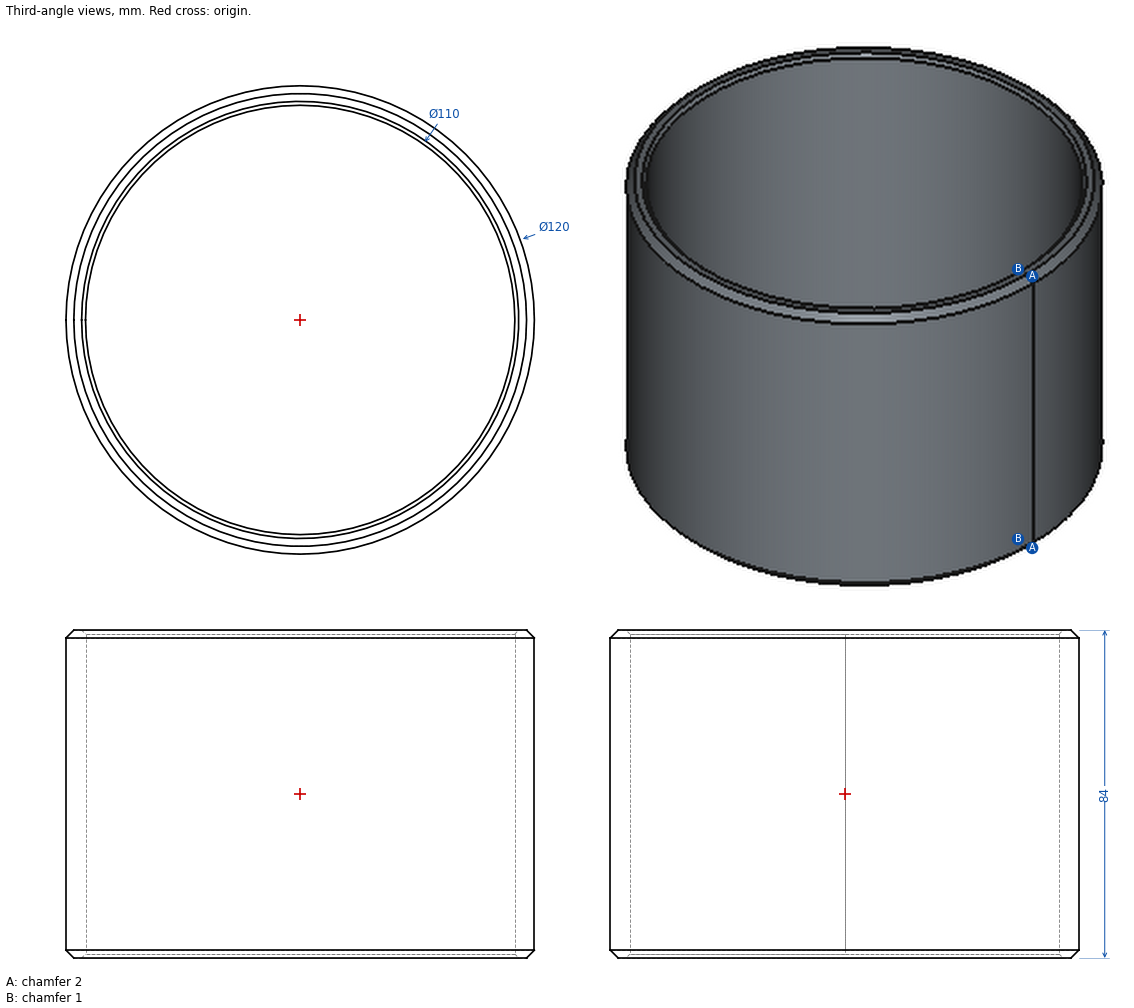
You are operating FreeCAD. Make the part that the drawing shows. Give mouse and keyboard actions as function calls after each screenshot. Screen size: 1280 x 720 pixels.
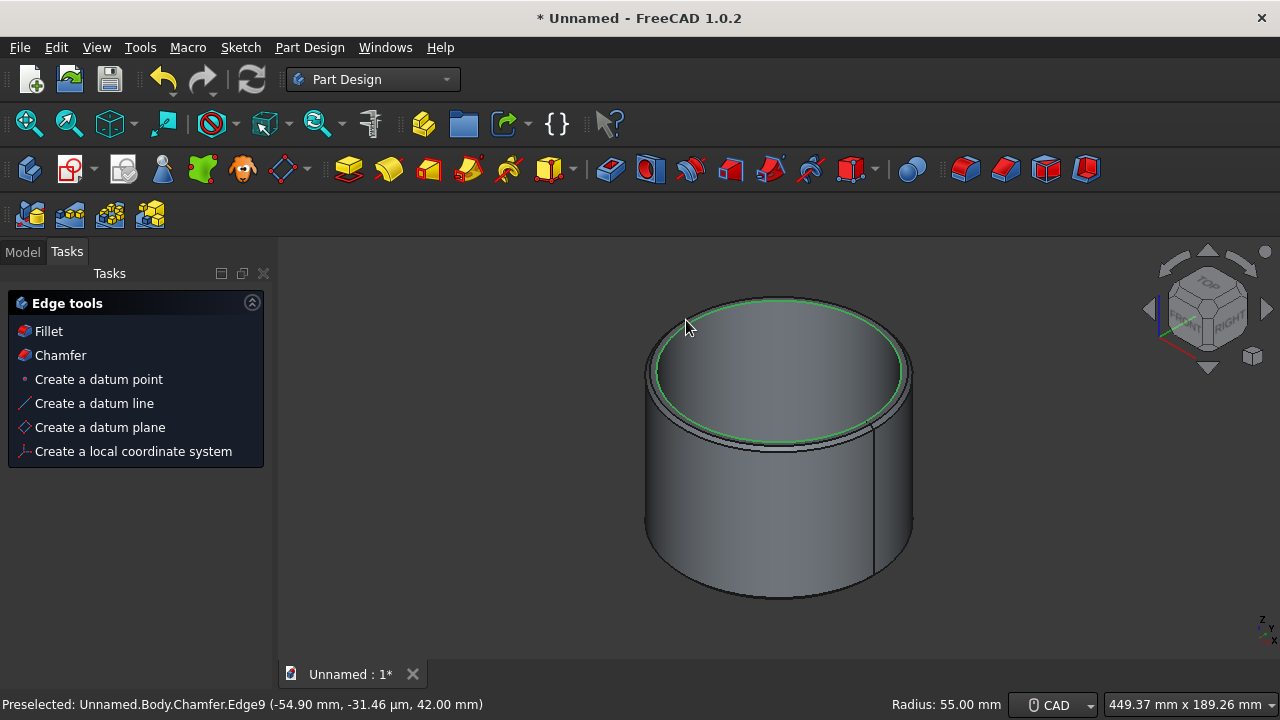
key(2)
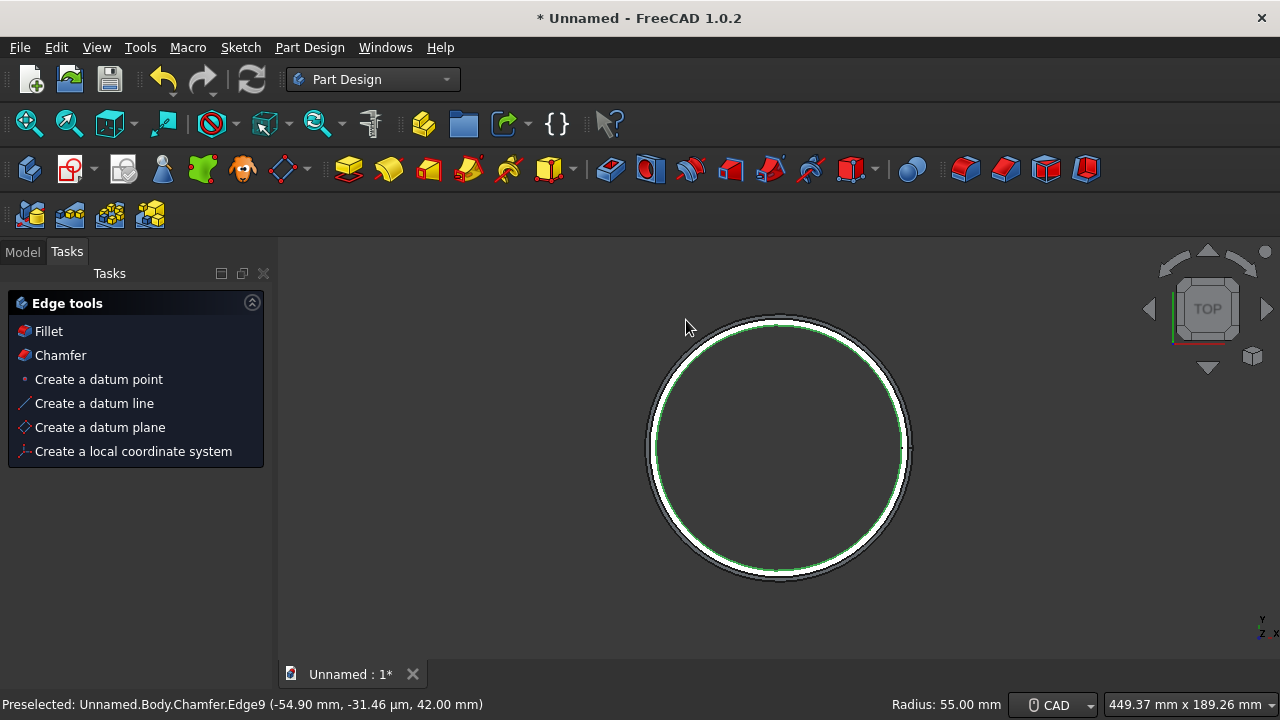
key(1)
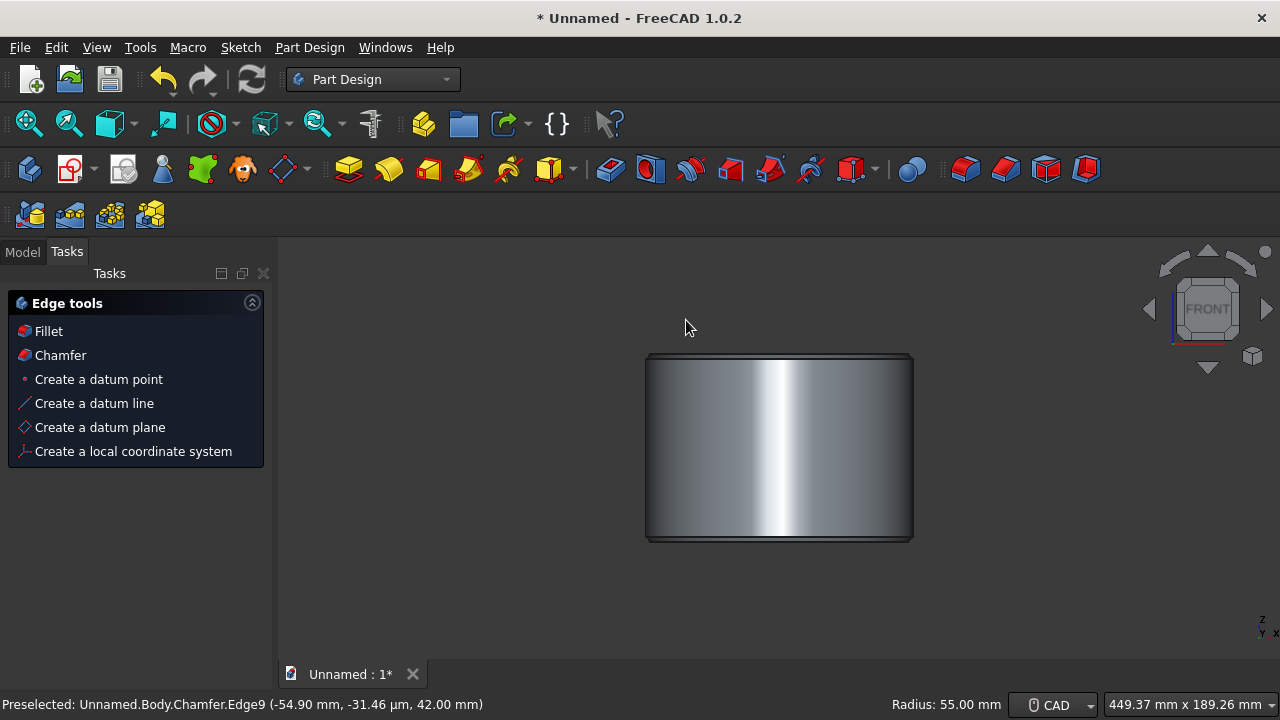
click(30, 124)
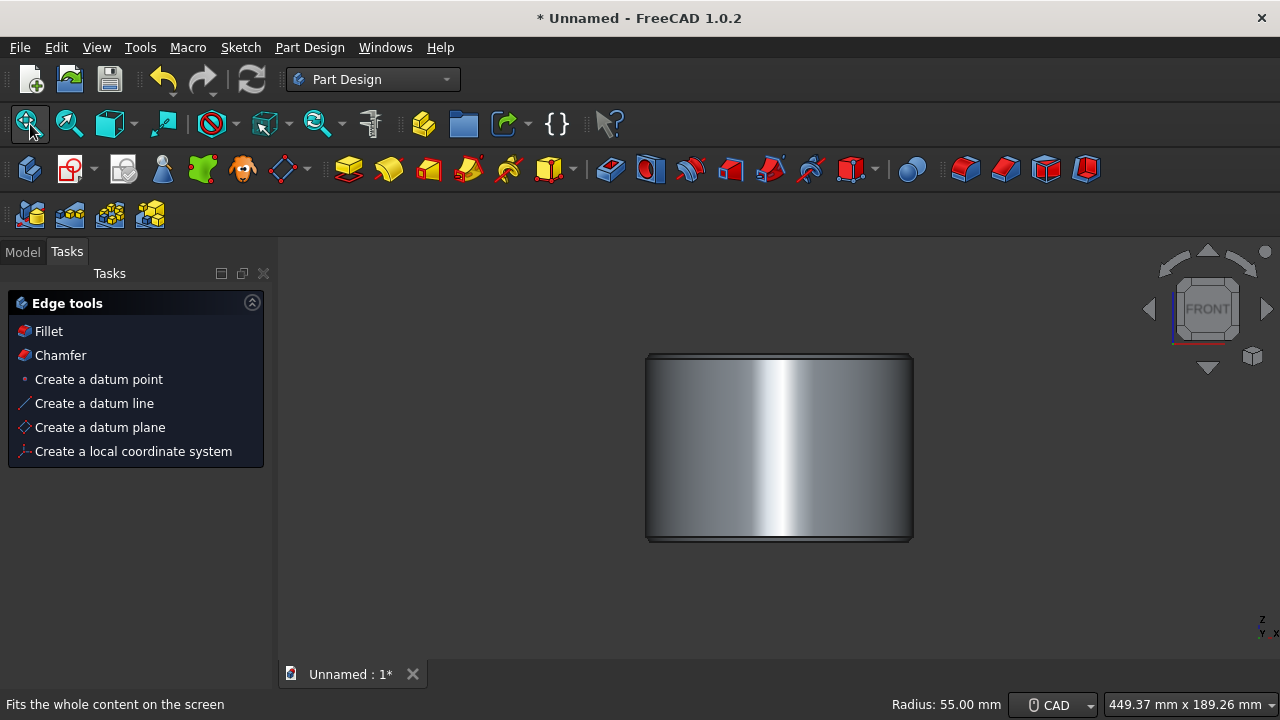
key(3)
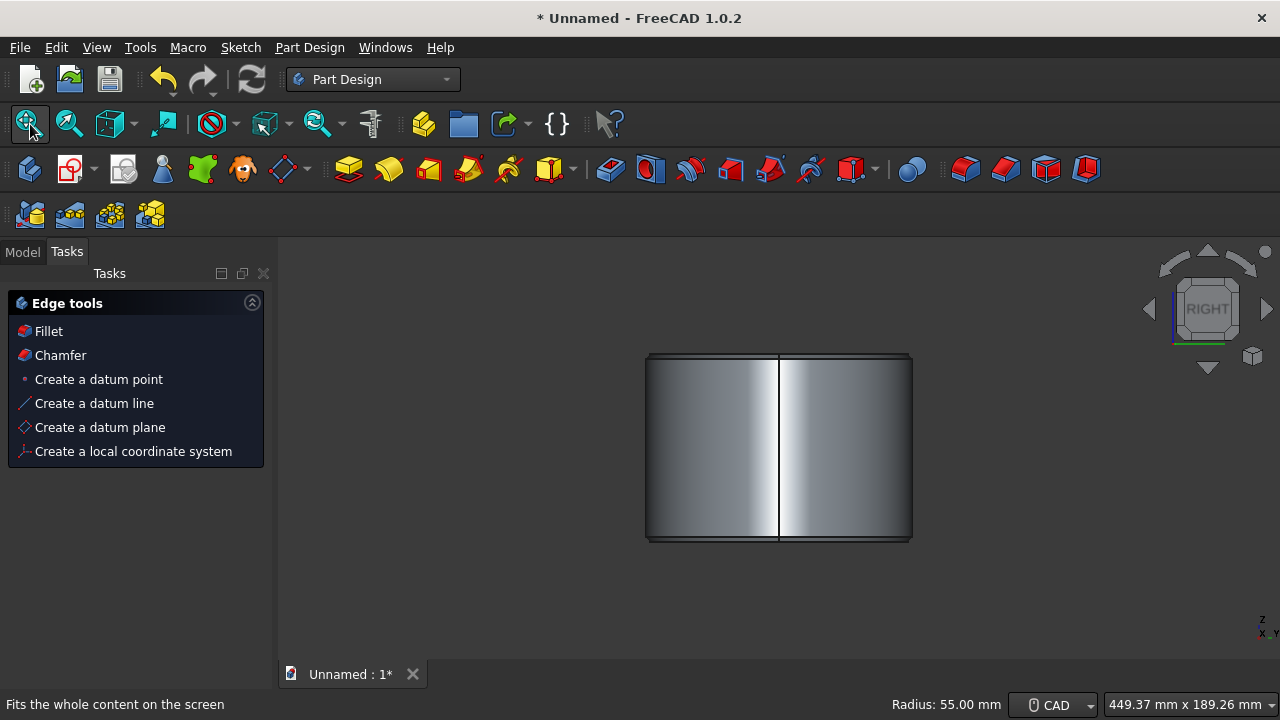
click(30, 124)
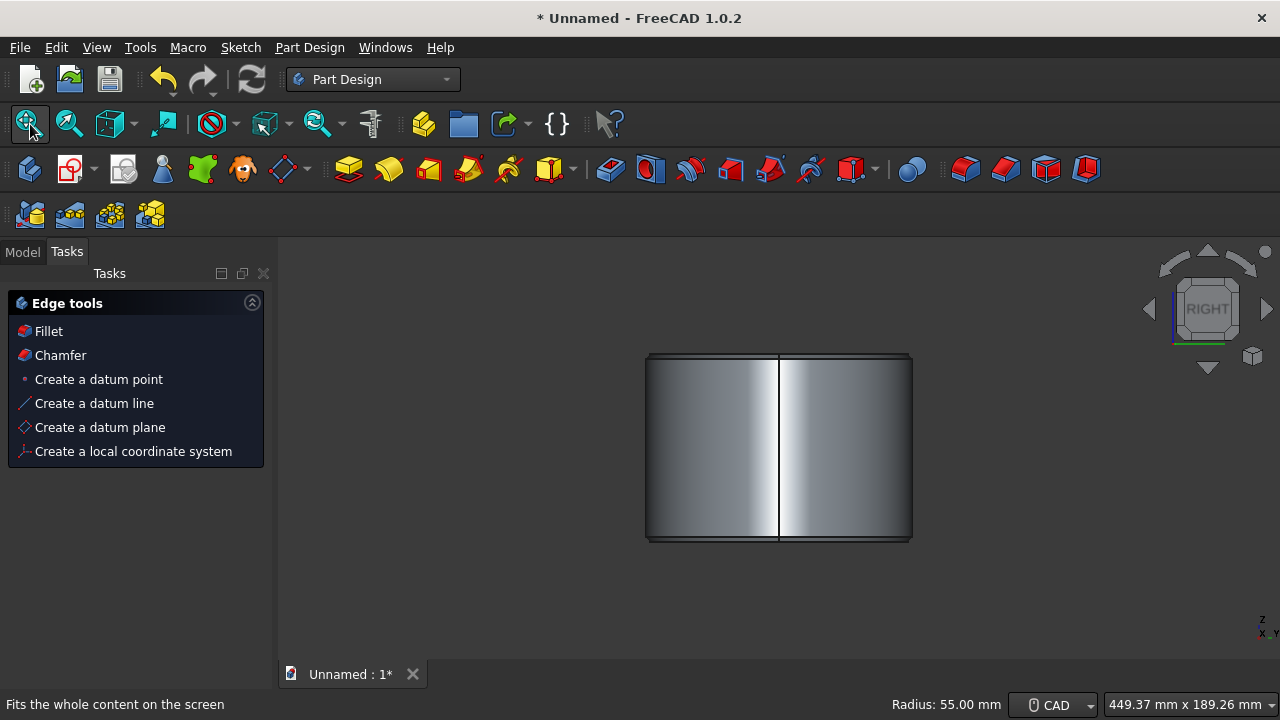
key(5)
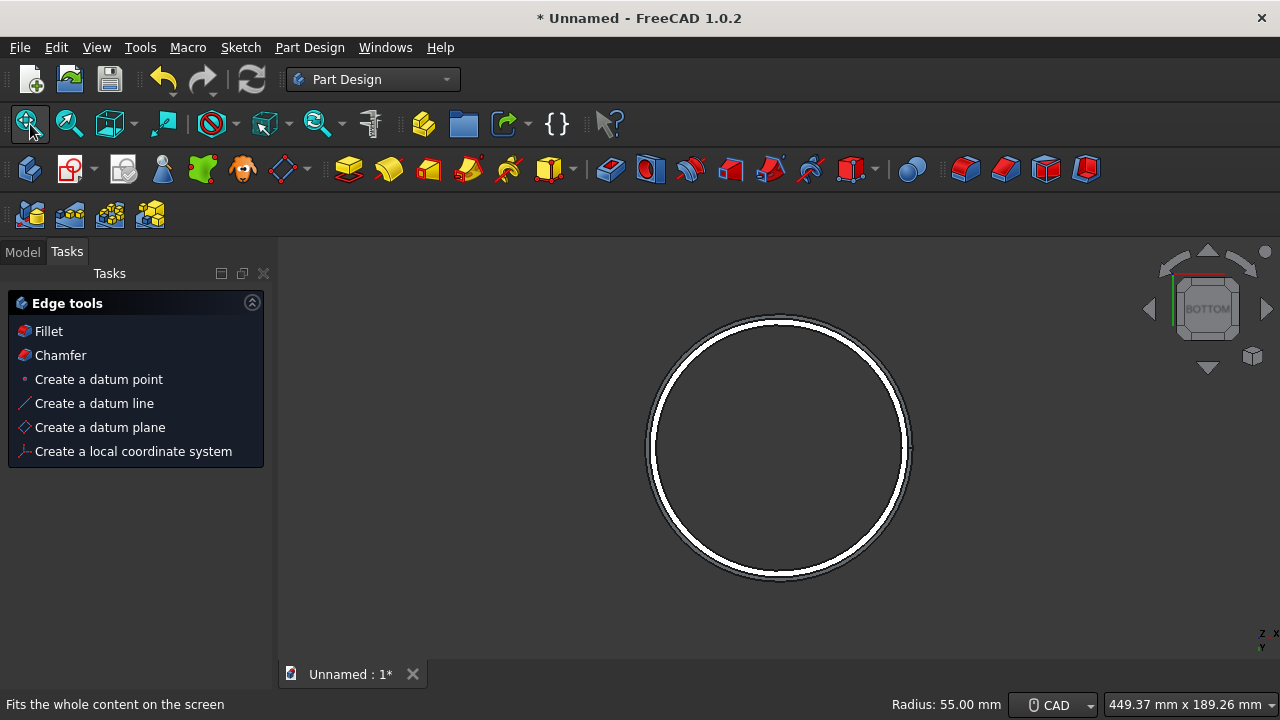
click(656, 447, ctrl)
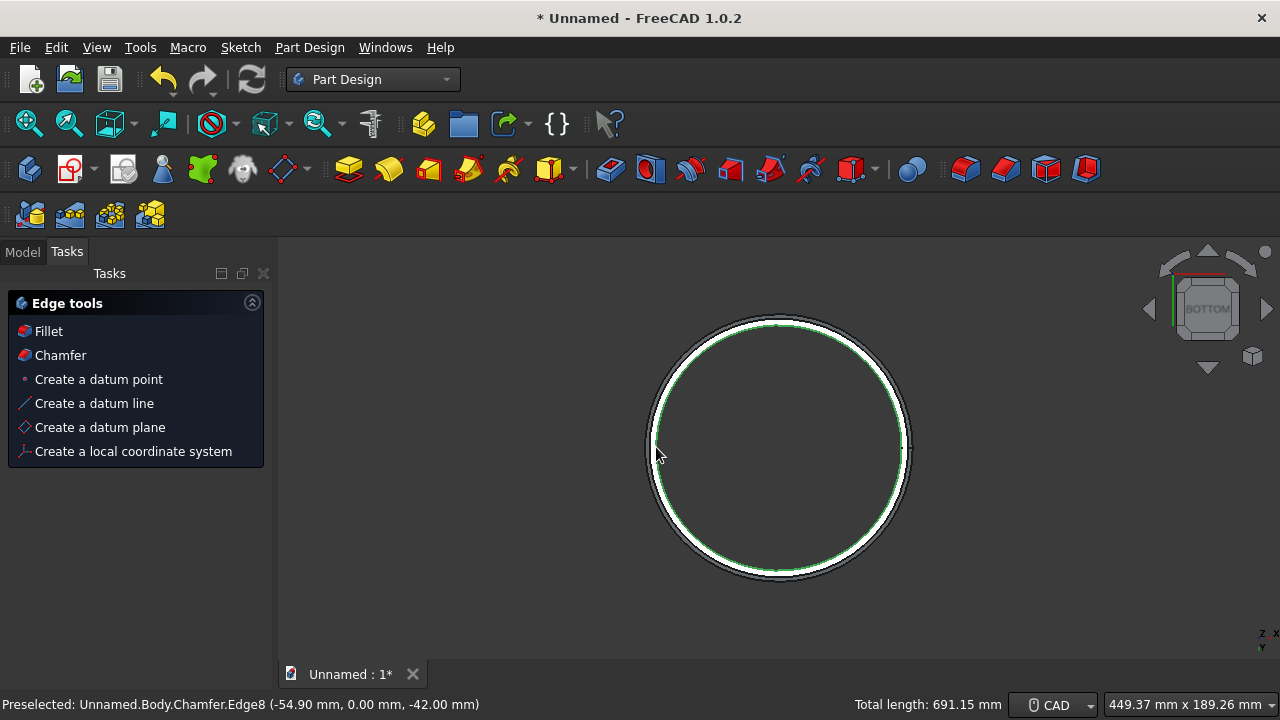
click(1006, 170)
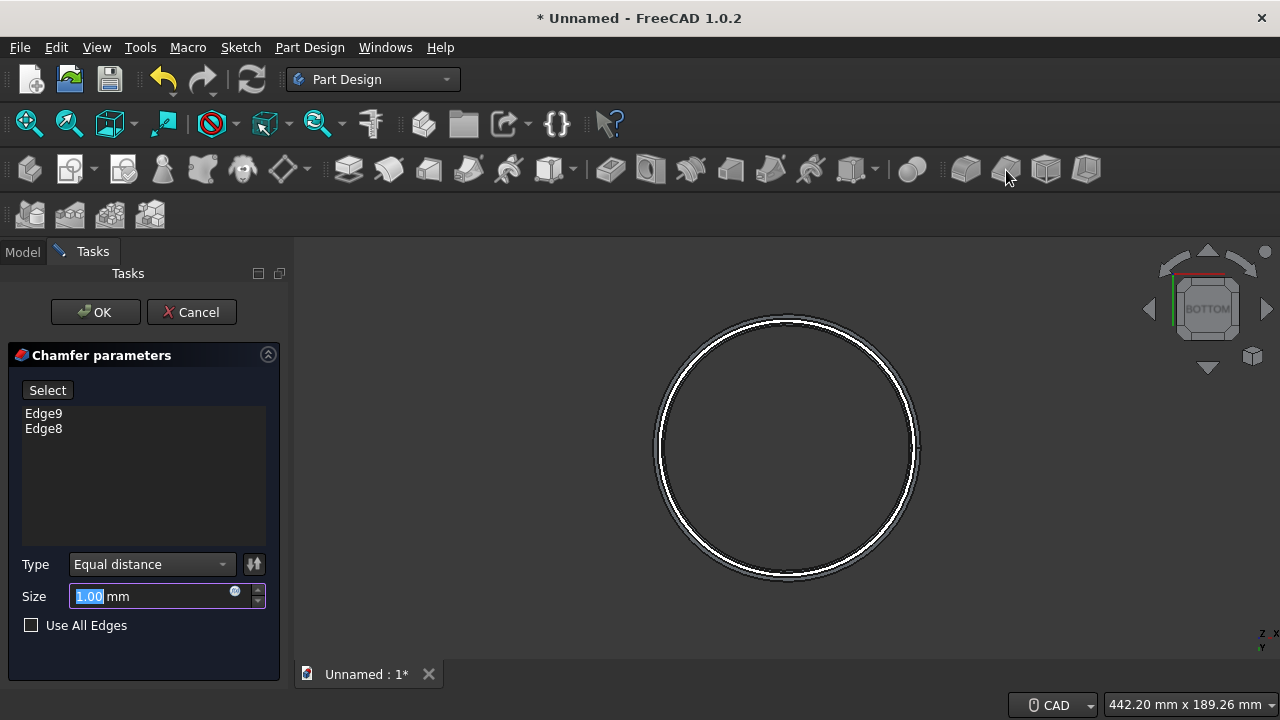
text(1)
key(Tab)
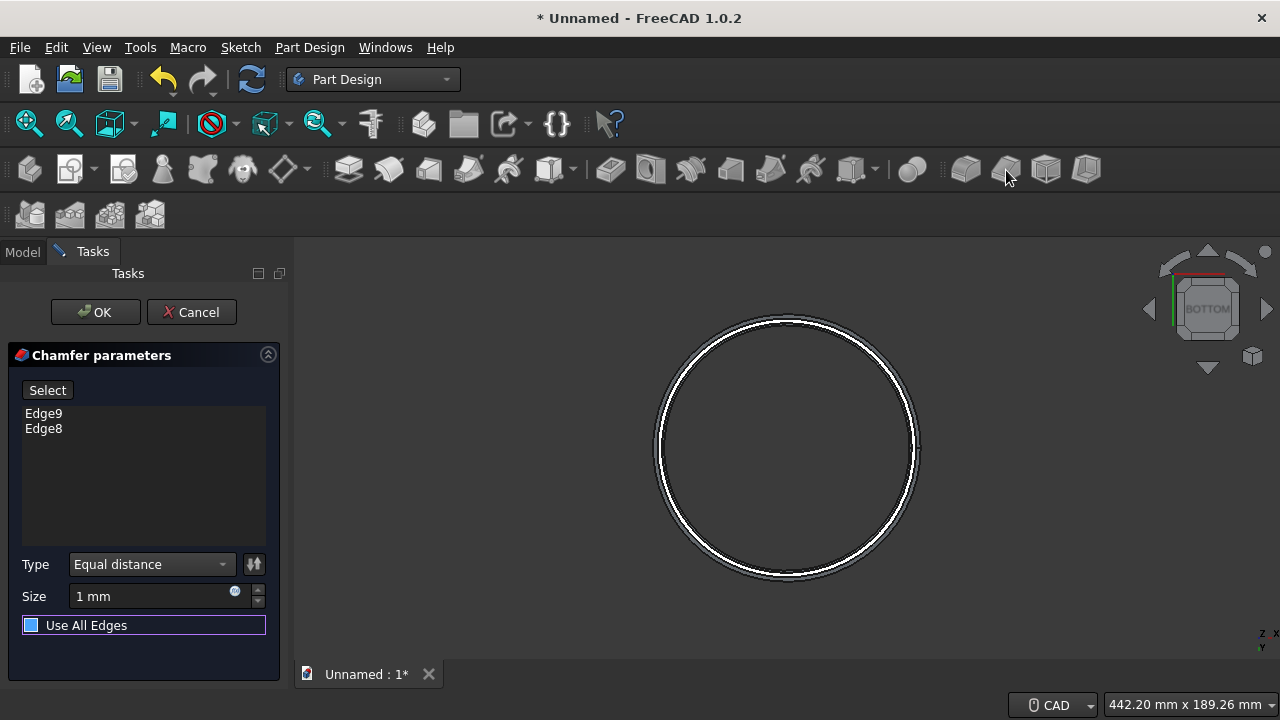
click(96, 312)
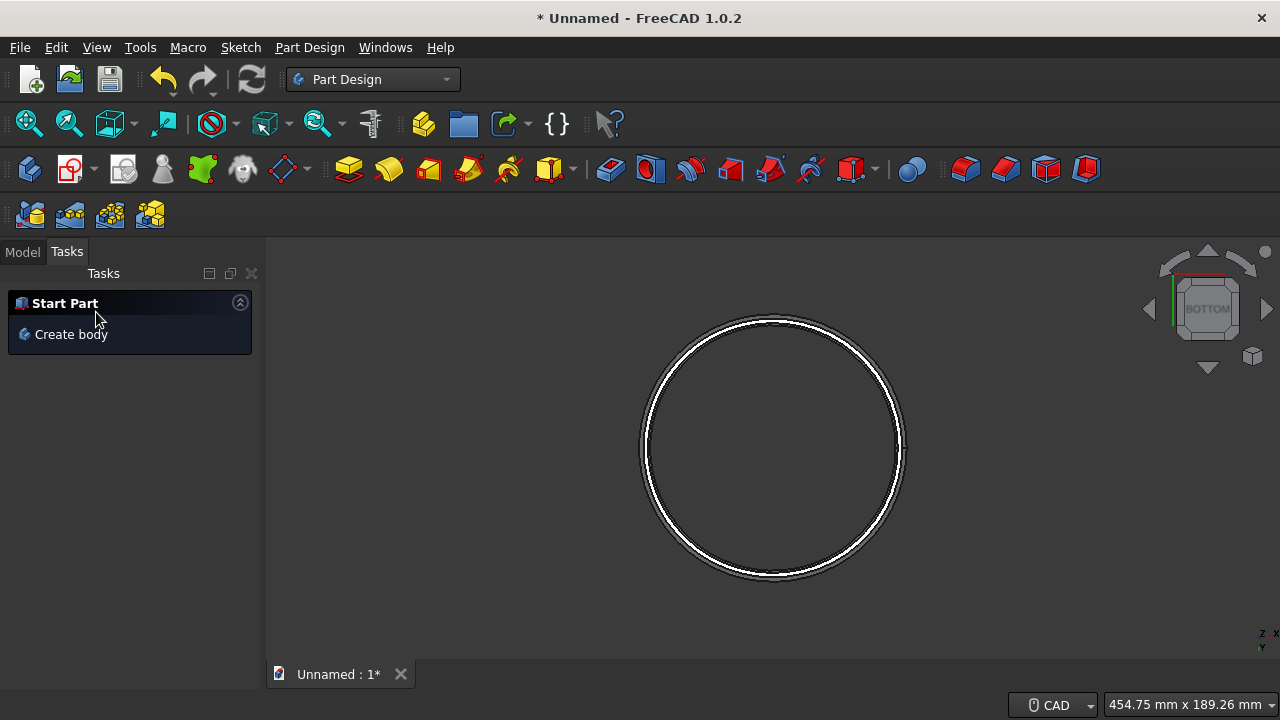
key(0)